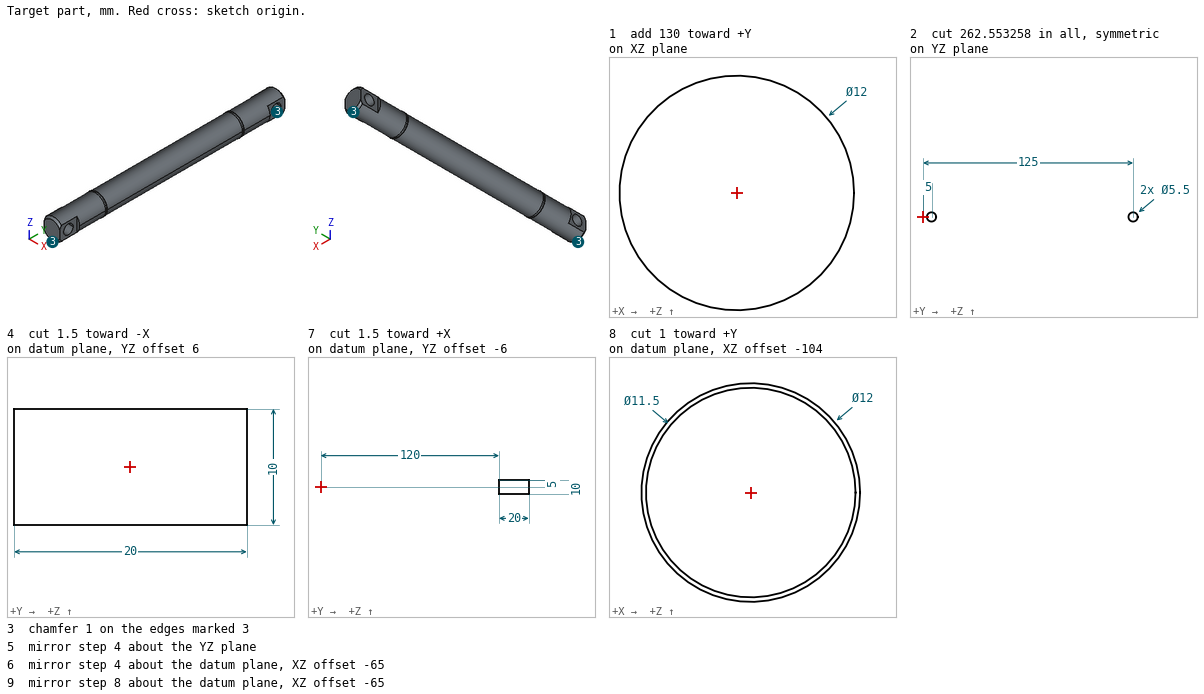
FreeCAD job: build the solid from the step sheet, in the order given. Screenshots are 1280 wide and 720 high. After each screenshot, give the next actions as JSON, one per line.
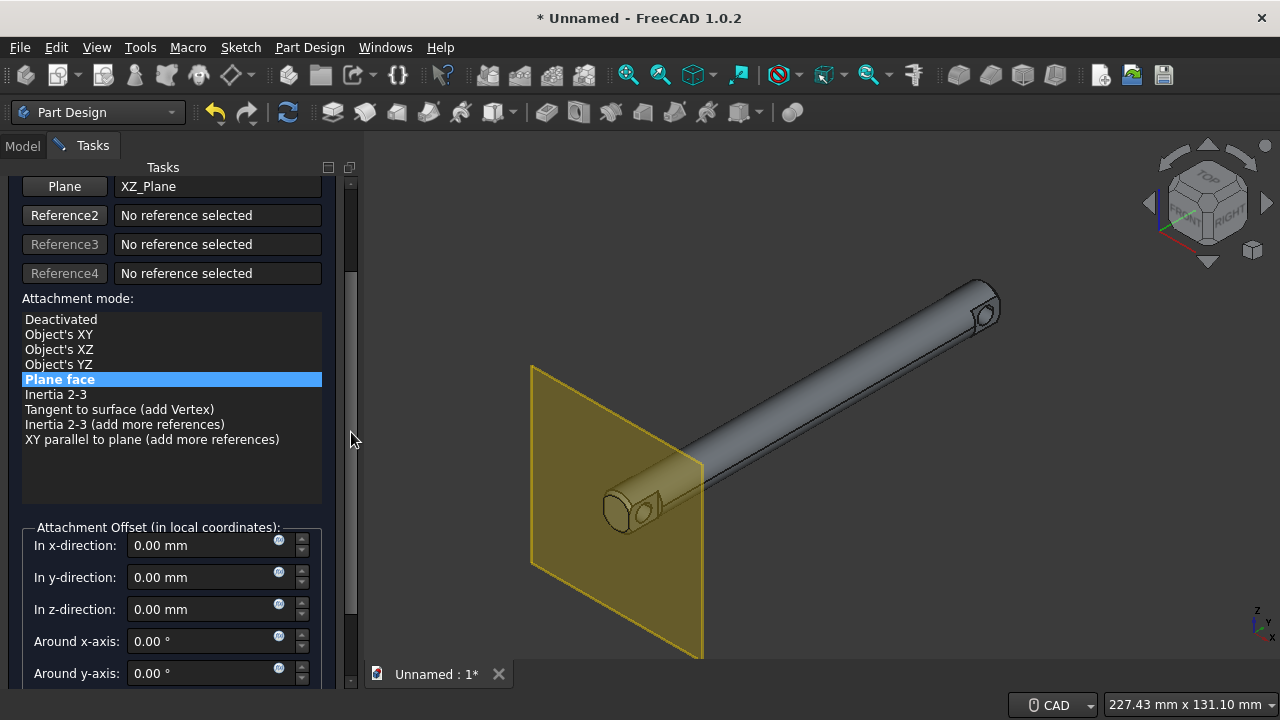
{"action": "triple_click", "coordinate": [210, 609]}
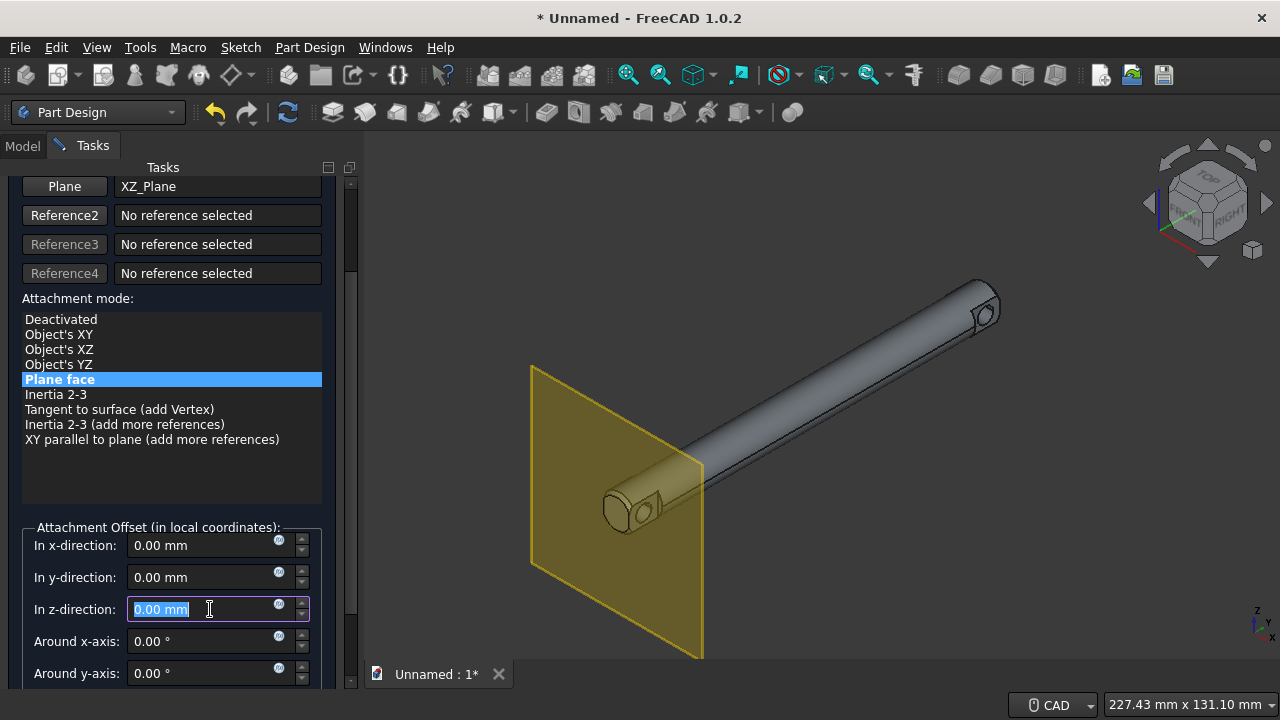
{"action": "type", "text": "-104"}
{"action": "key", "text": "Tab"}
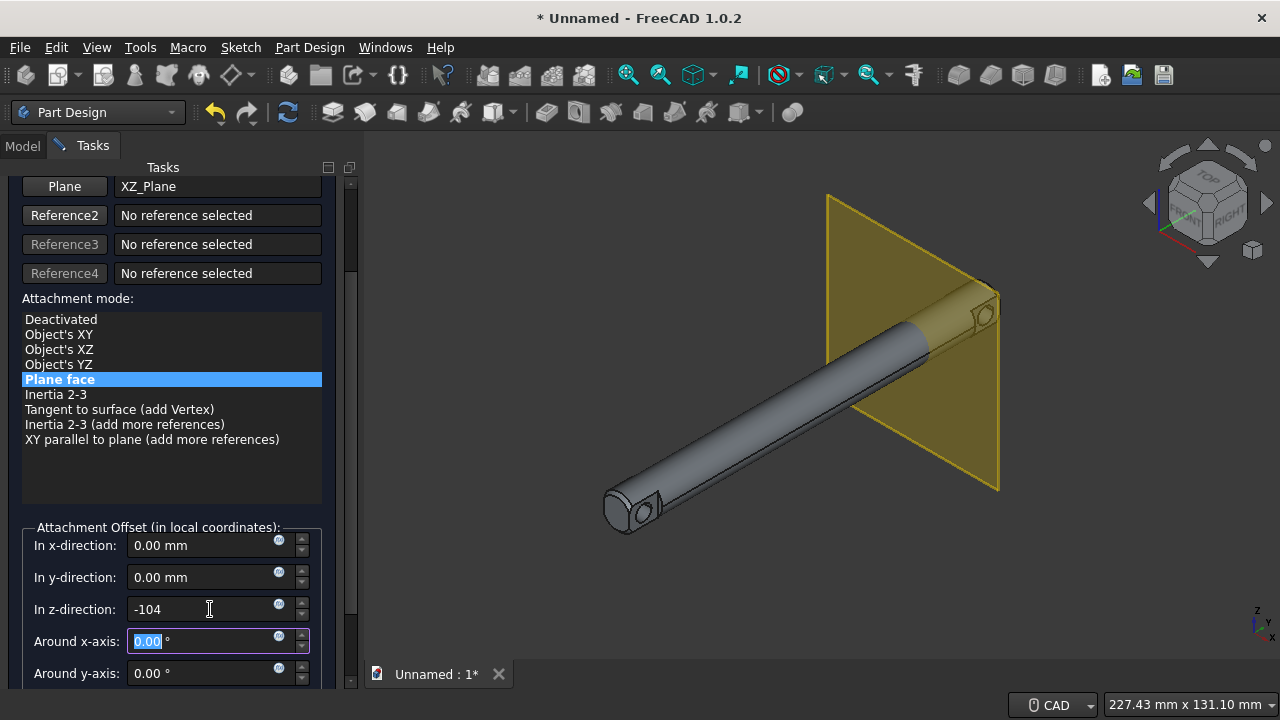
{"action": "scroll", "coordinate": [351, 432], "scroll_direction": "up", "scroll_amount": 3}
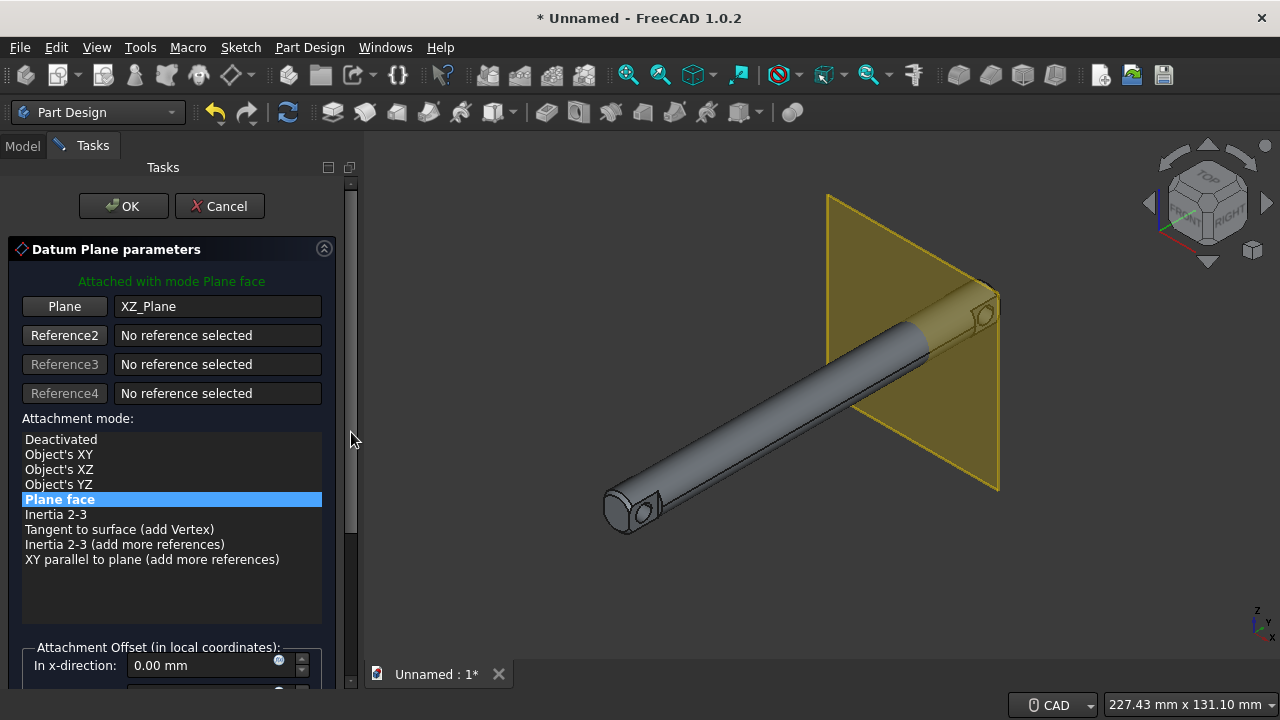
{"action": "left_click", "coordinate": [124, 206]}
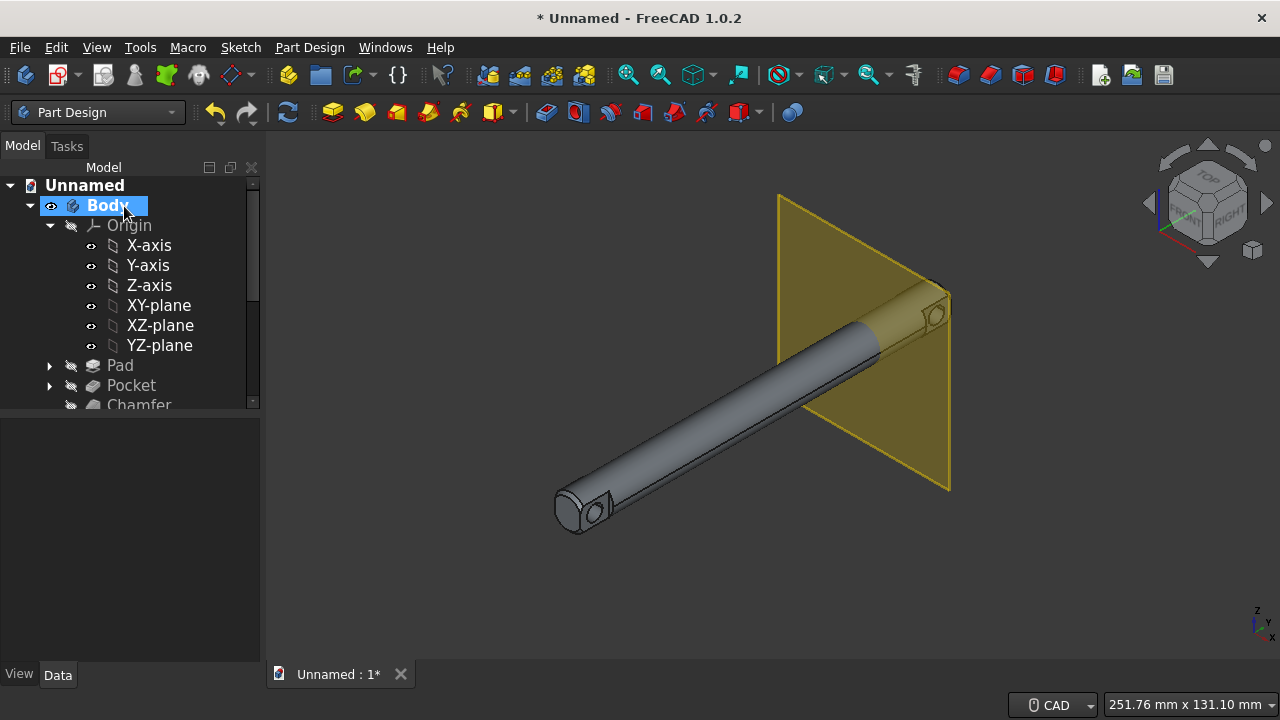
{"action": "scroll", "coordinate": [100, 301], "scroll_direction": "down", "scroll_amount": 3}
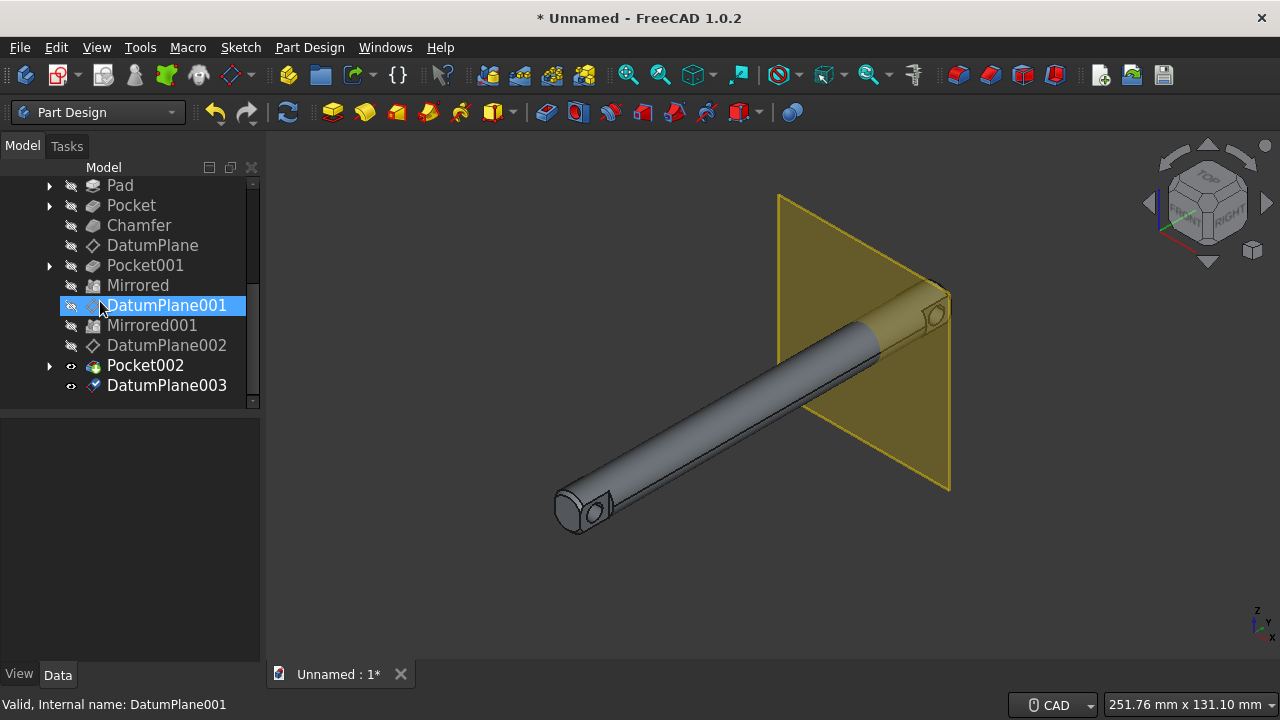
{"action": "left_click", "coordinate": [116, 386]}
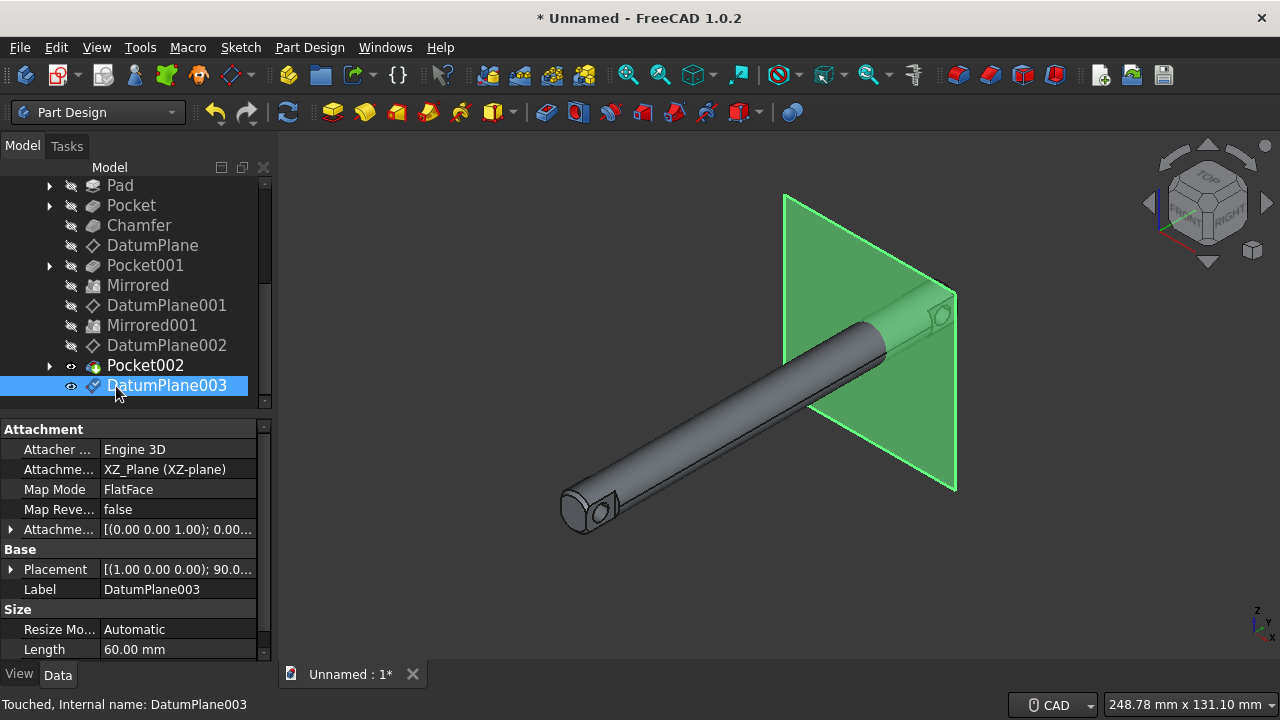
{"action": "left_click", "coordinate": [58, 76]}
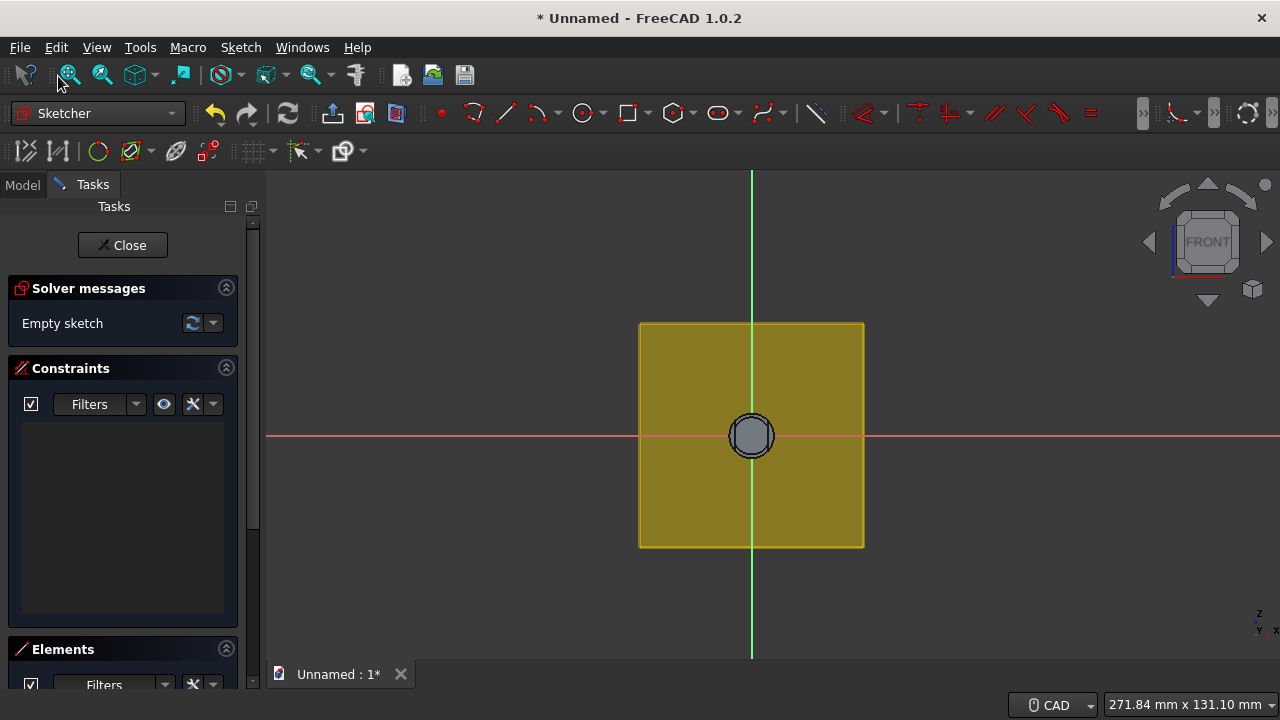
{"action": "key", "text": "q s"}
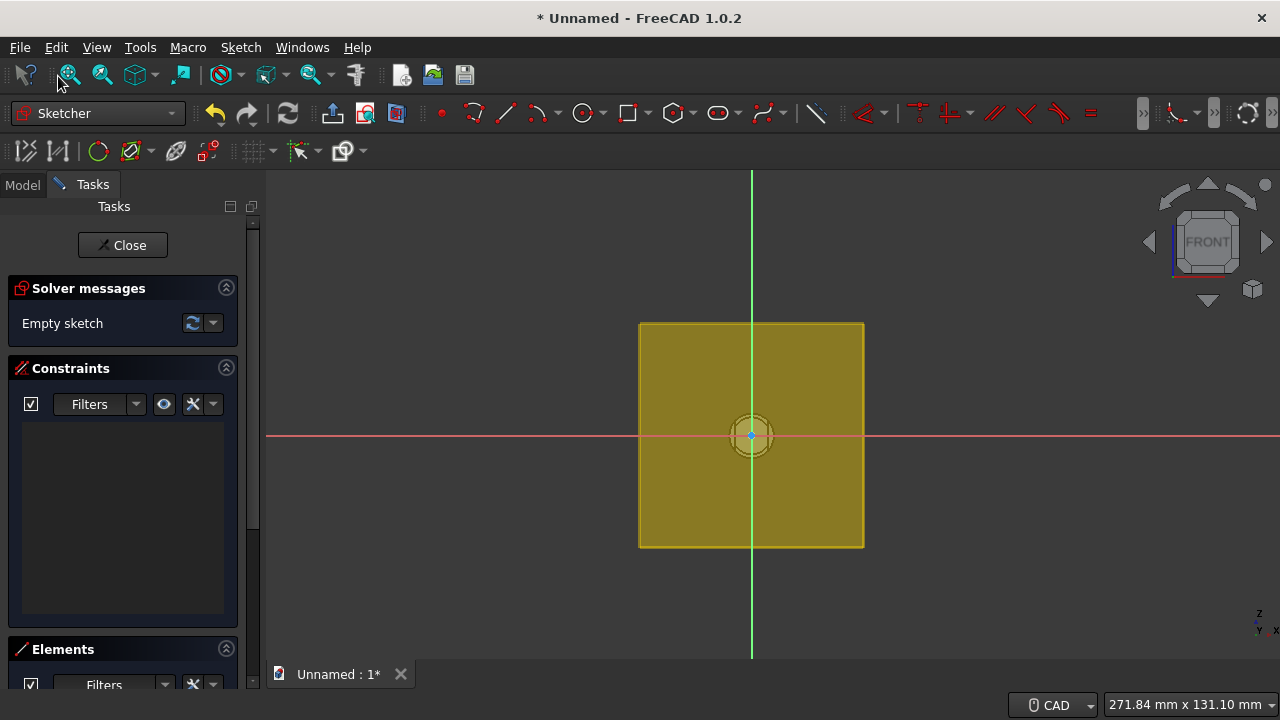
{"action": "scroll", "coordinate": [759, 439], "scroll_direction": "up", "scroll_amount": 10}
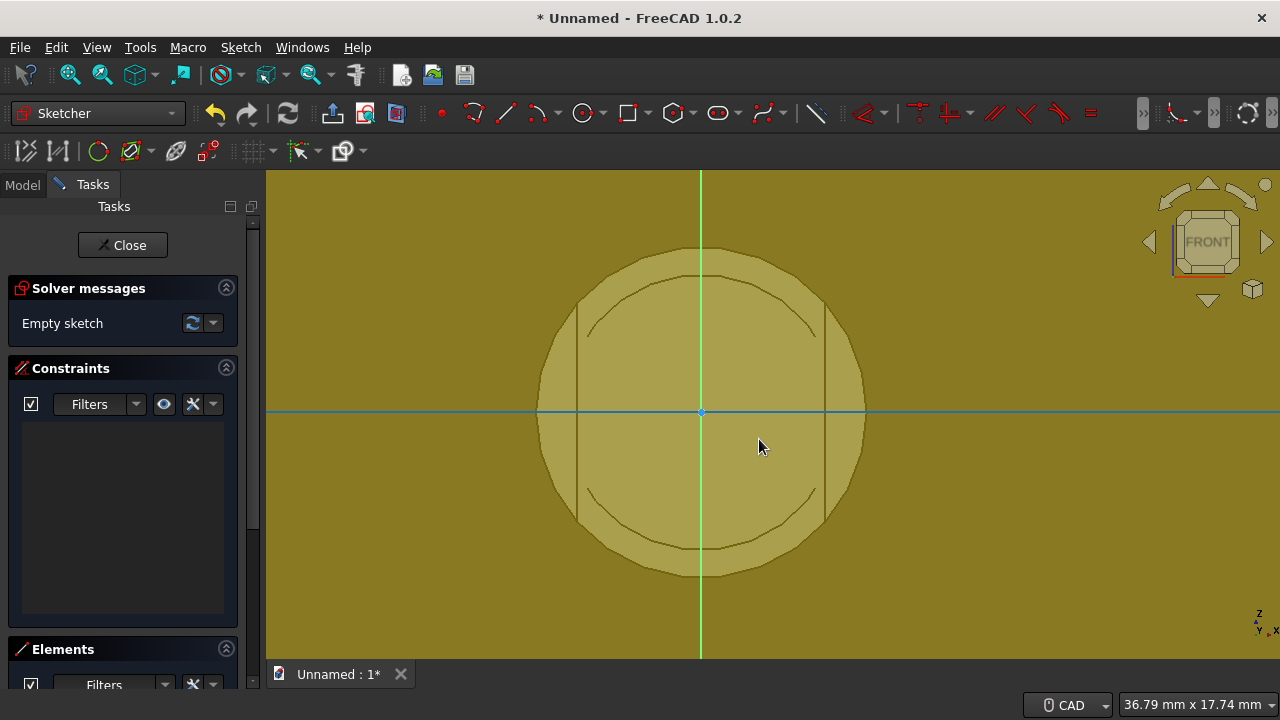
{"action": "key", "text": "g c"}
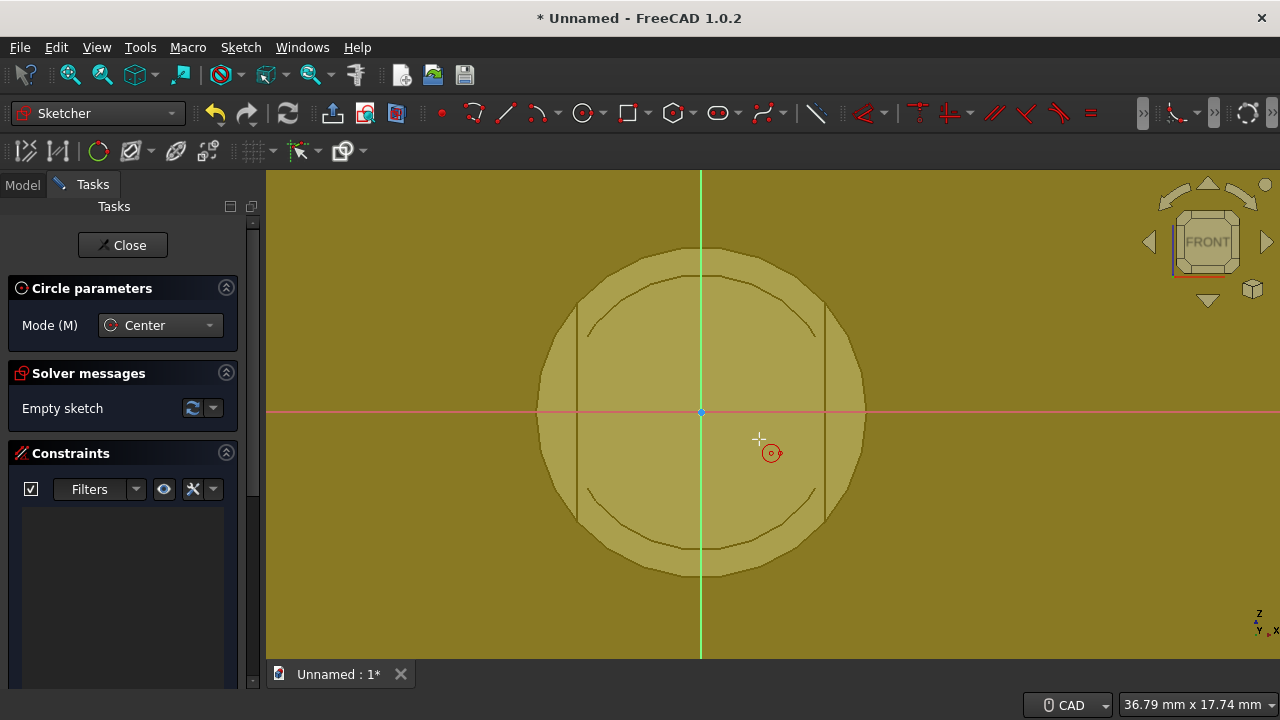
{"action": "left_click", "coordinate": [701, 412]}
{"action": "mouse_move", "coordinate": [818, 296]}